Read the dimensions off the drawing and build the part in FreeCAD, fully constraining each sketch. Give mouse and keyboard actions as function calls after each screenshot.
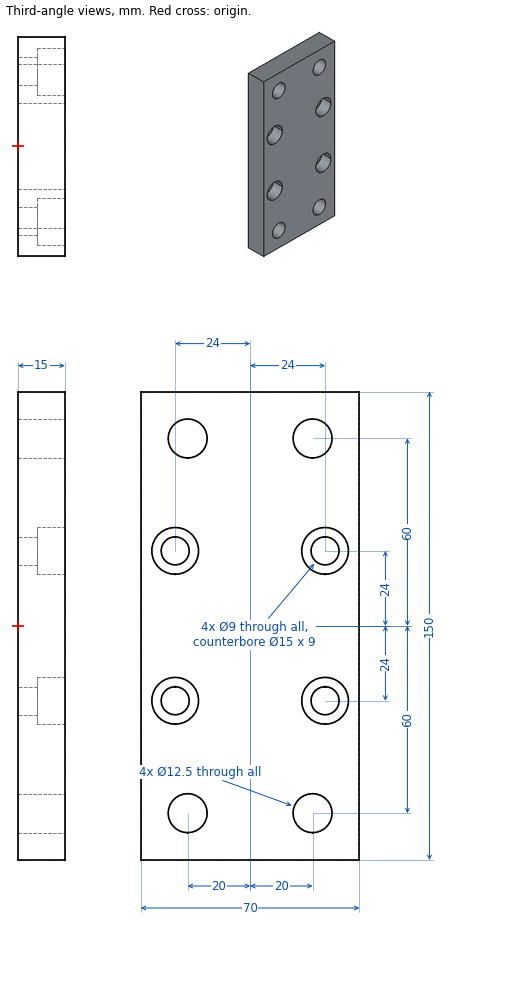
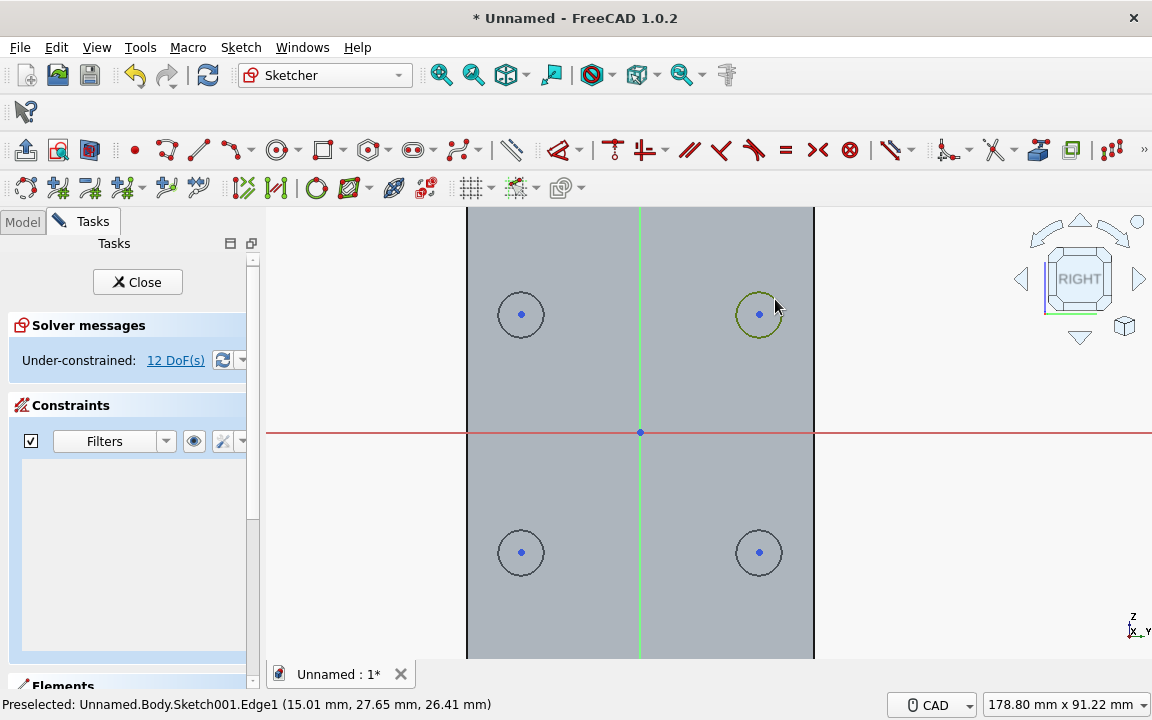
click(775, 537)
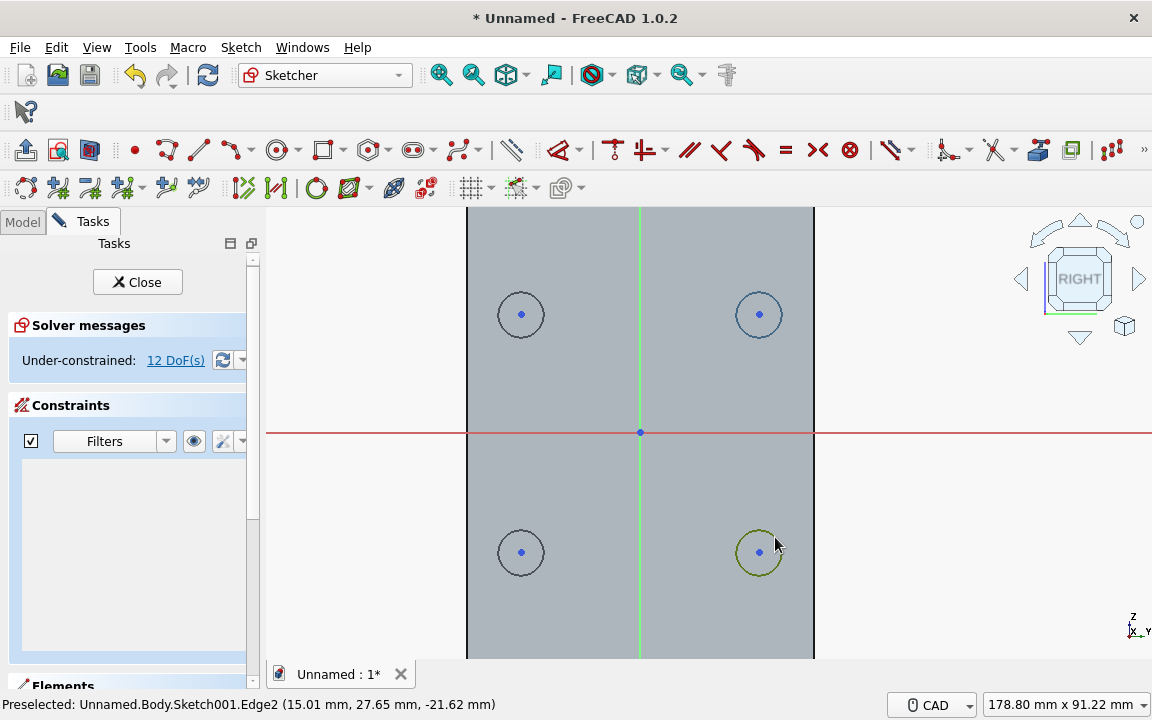
click(537, 299)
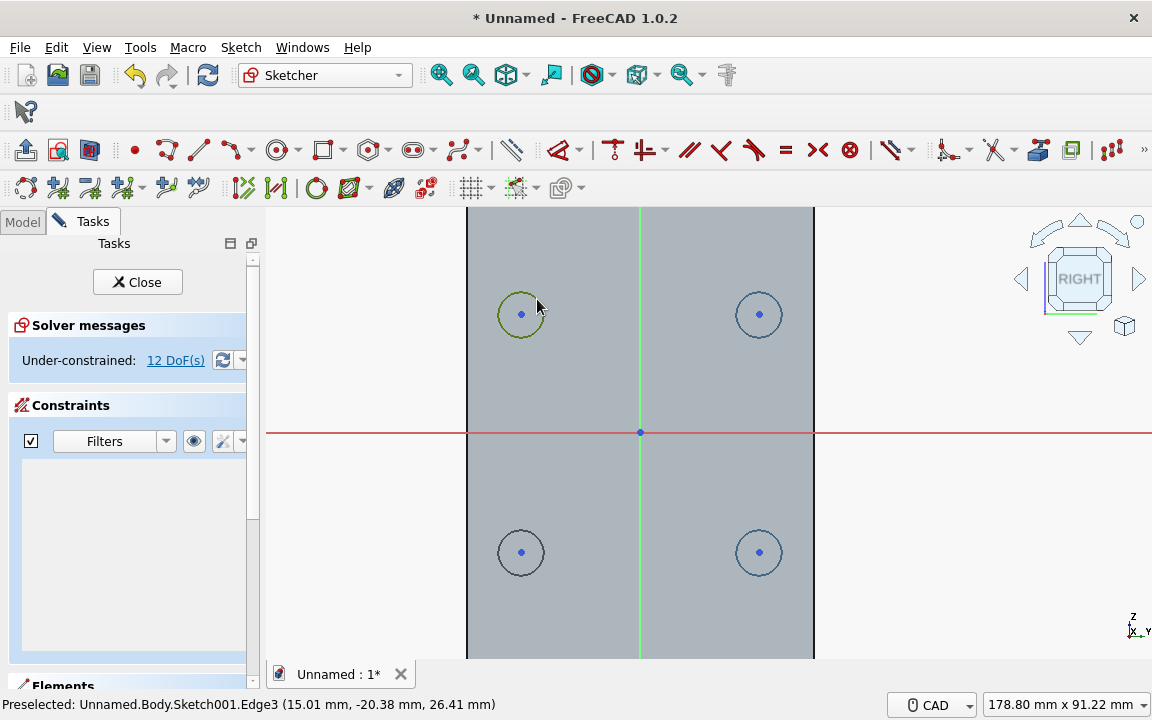
click(537, 537)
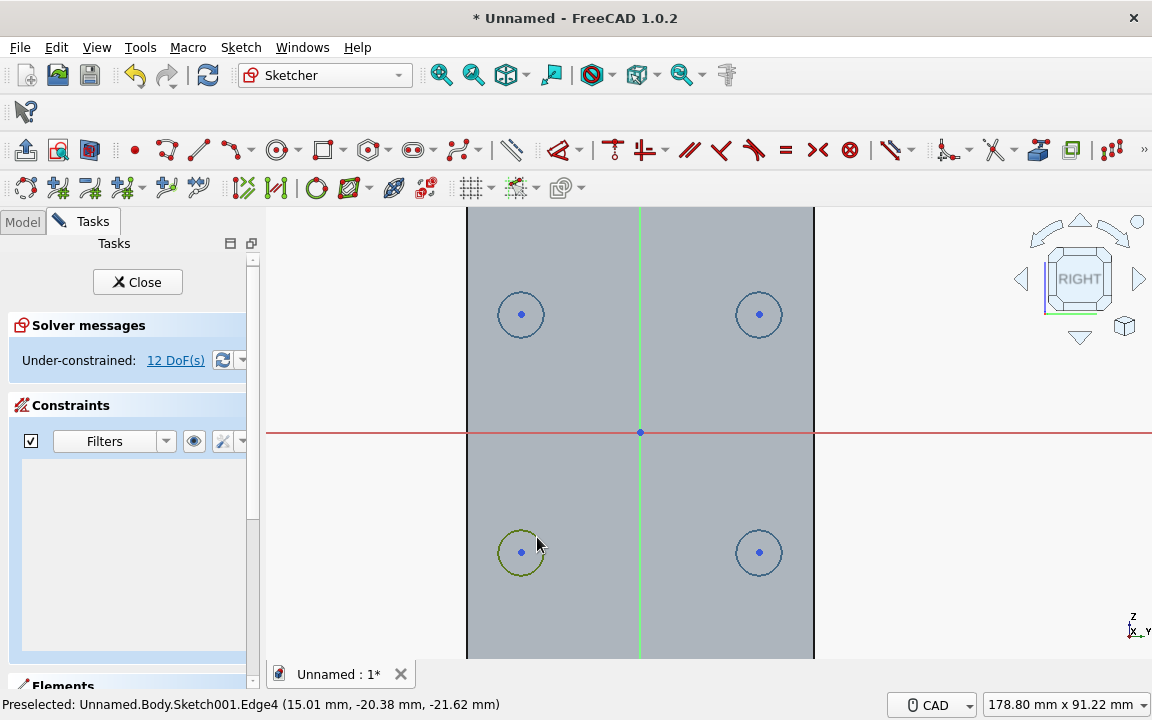
click(786, 150)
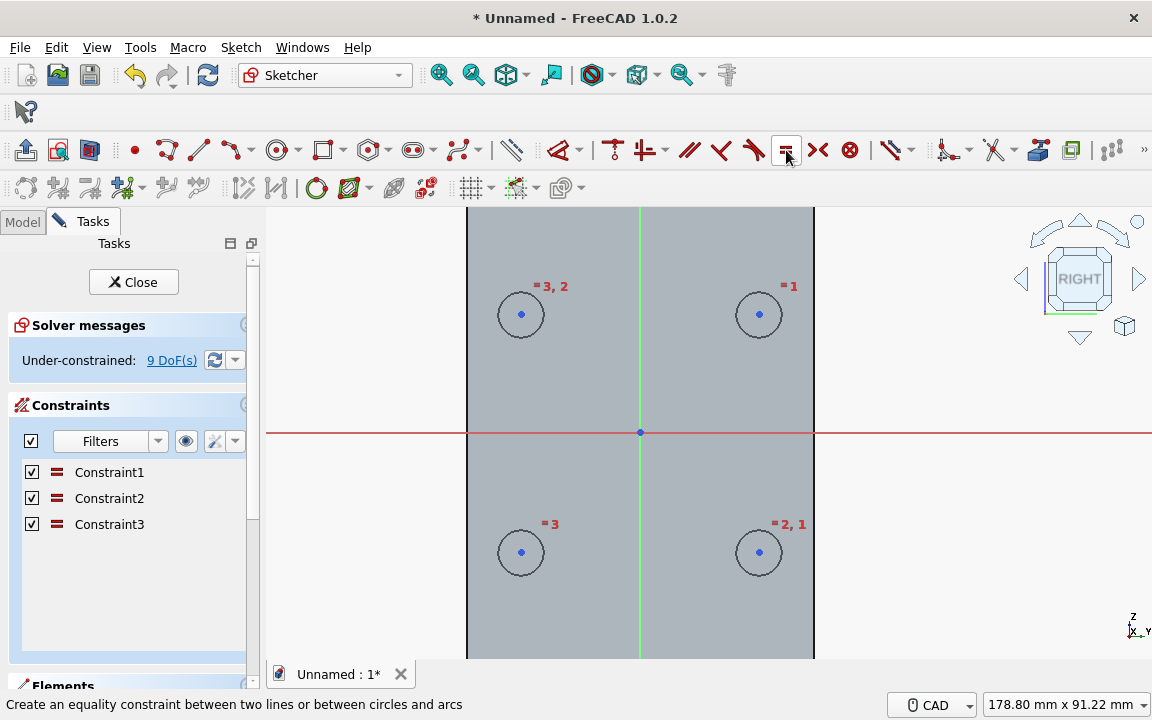
click(759, 315)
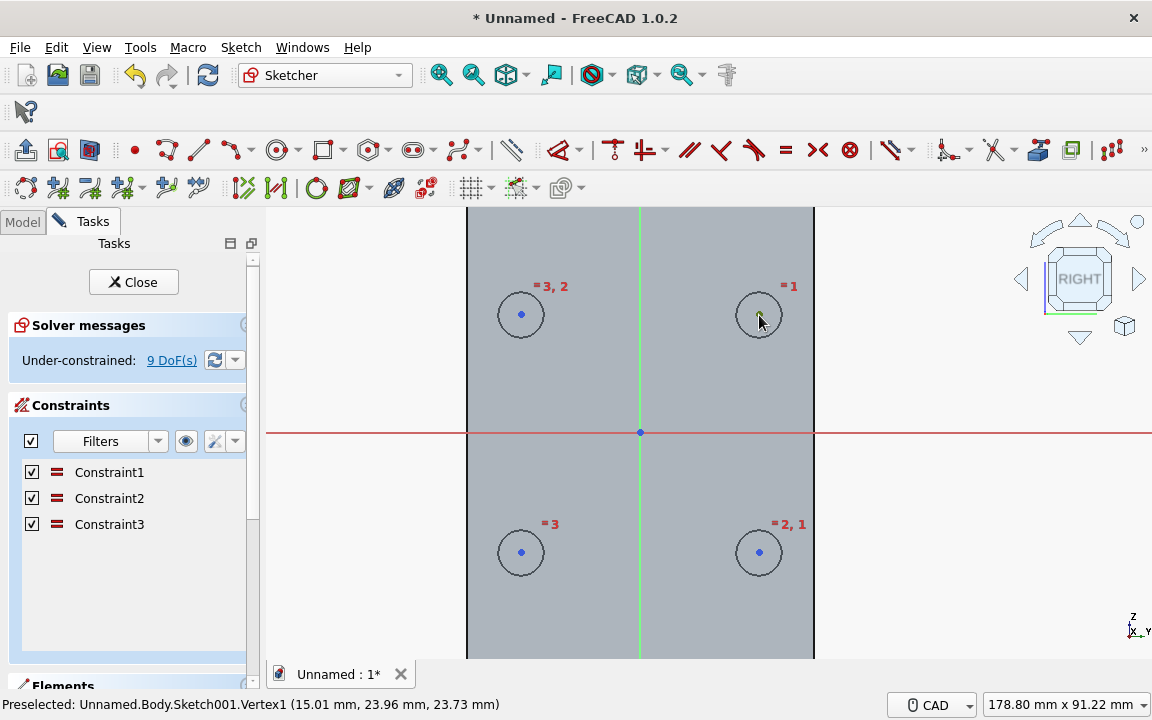
click(759, 553)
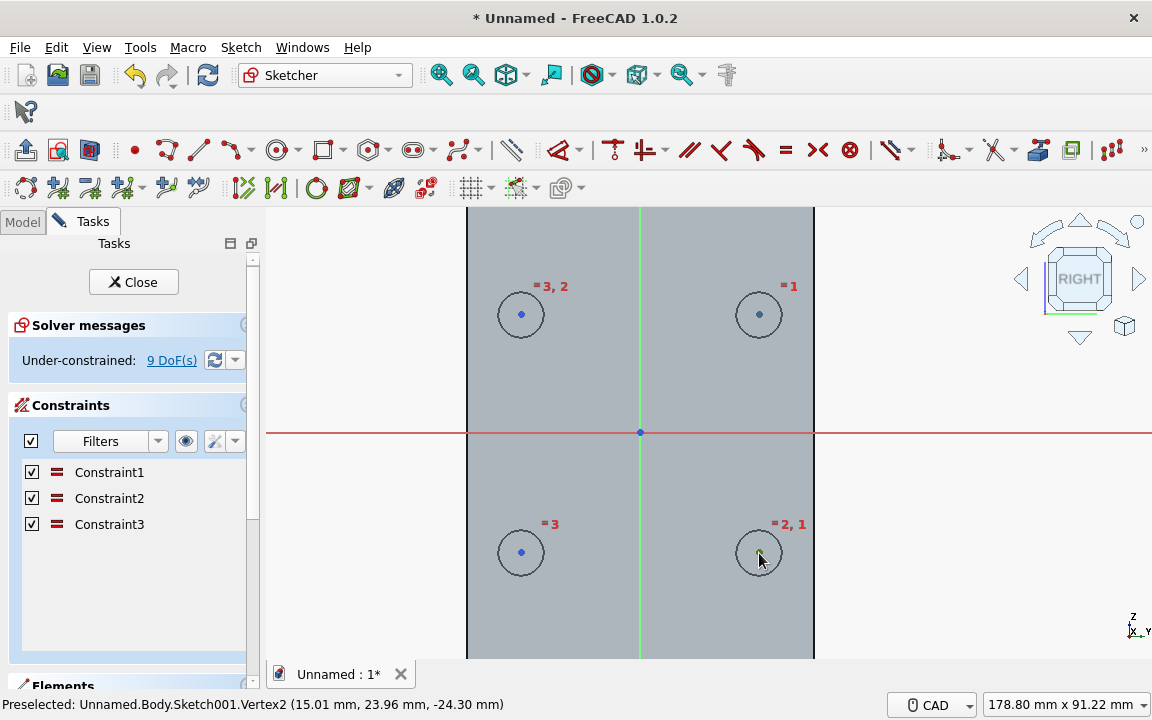
key(v)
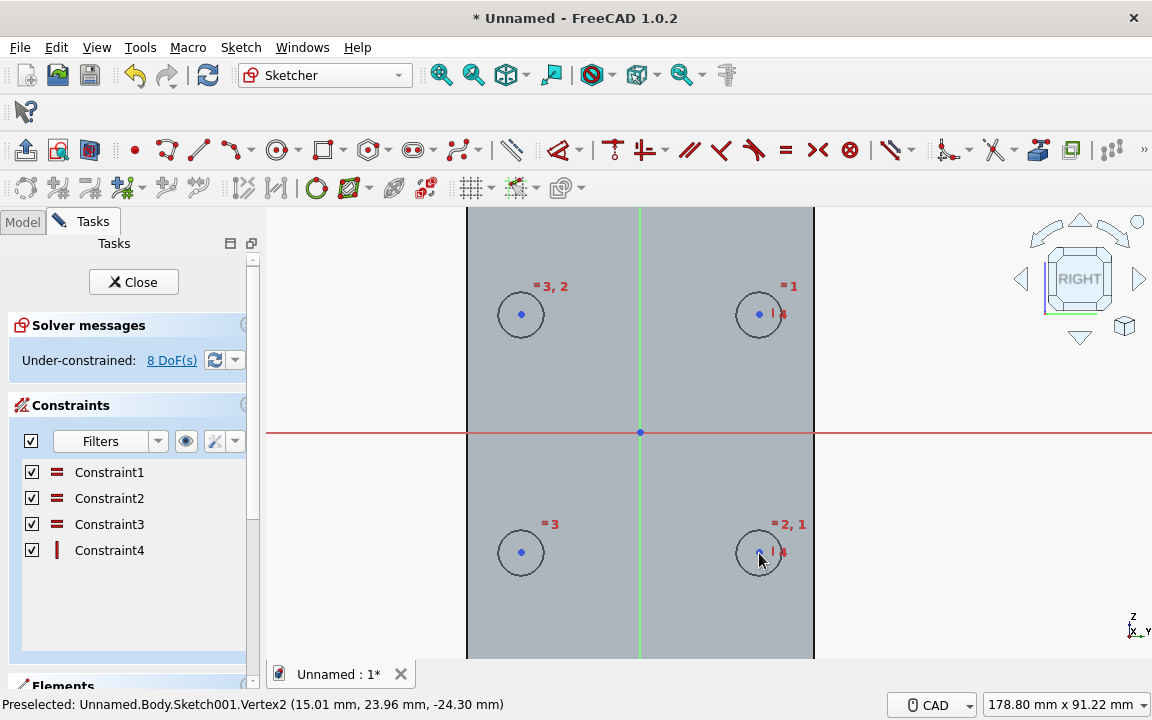
click(759, 315)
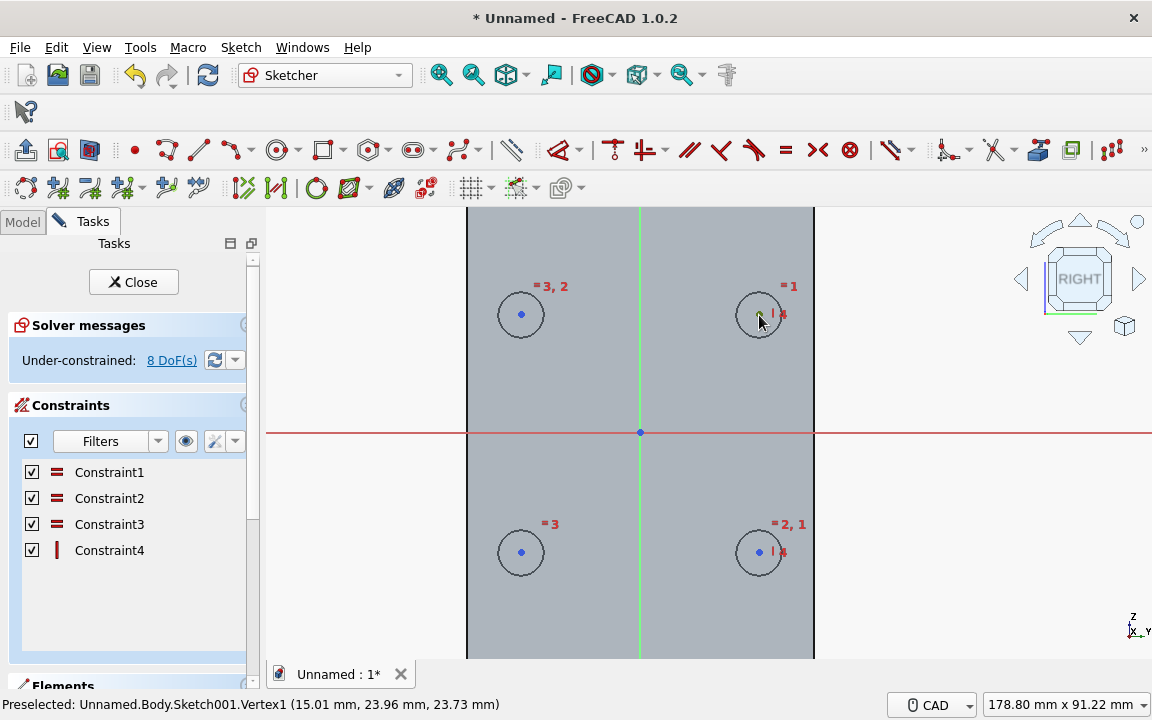
click(521, 315)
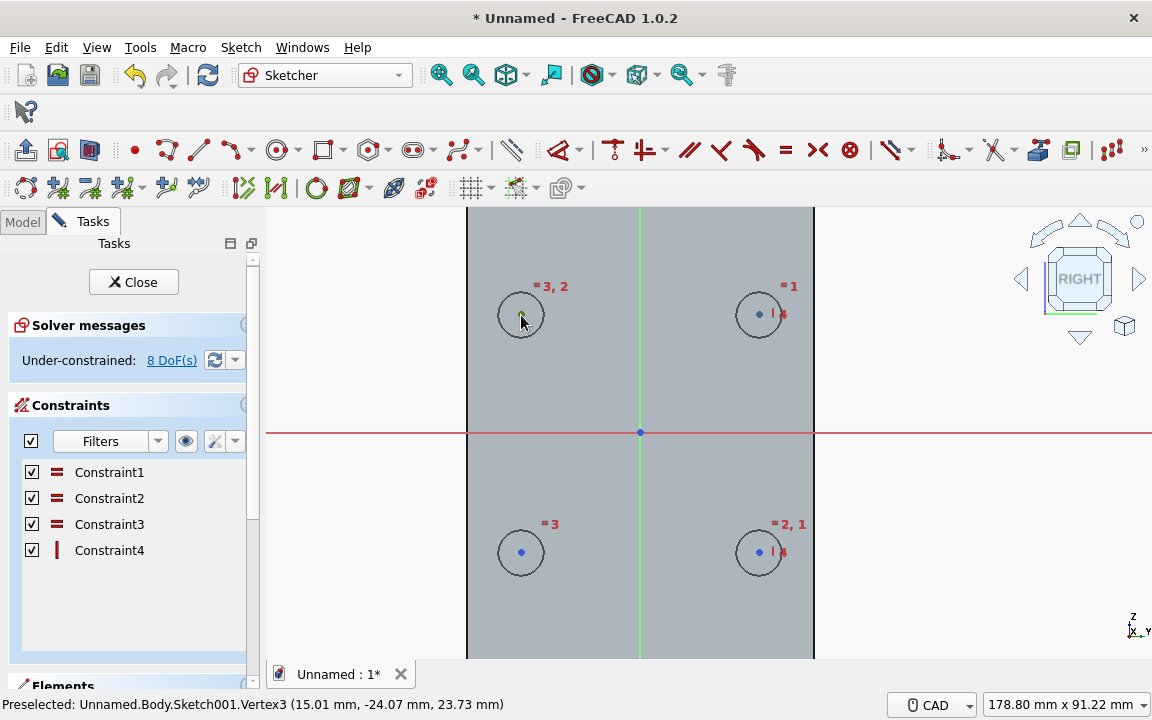
click(668, 150)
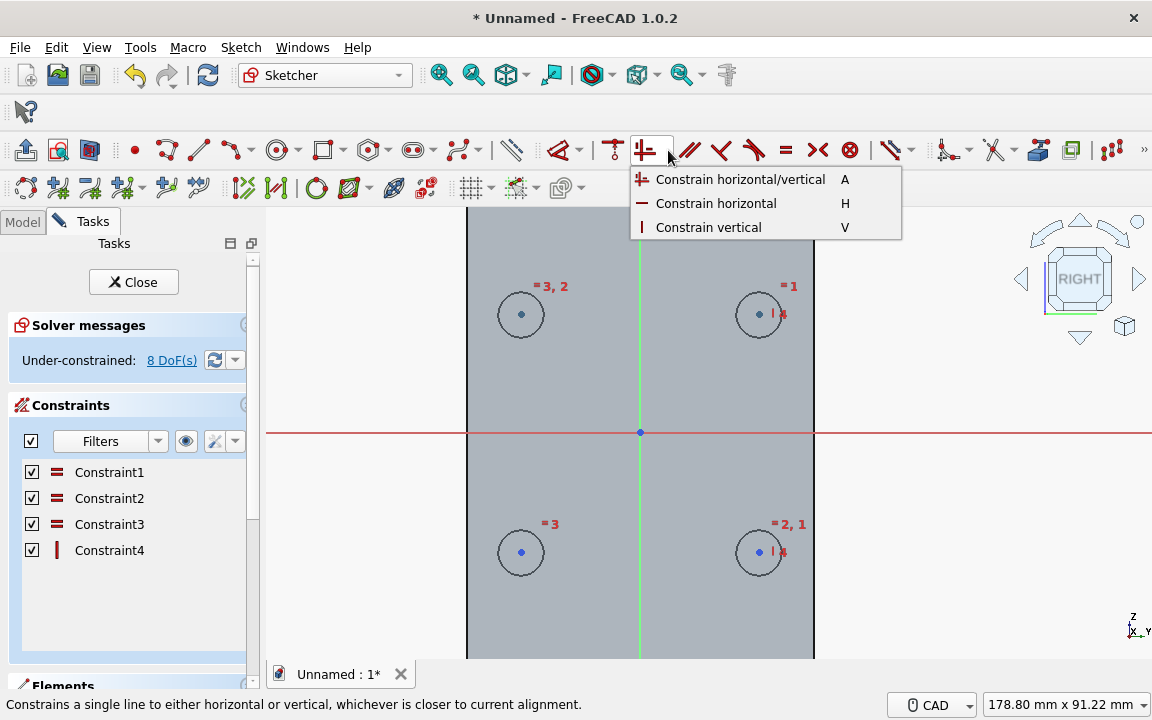
click(766, 203)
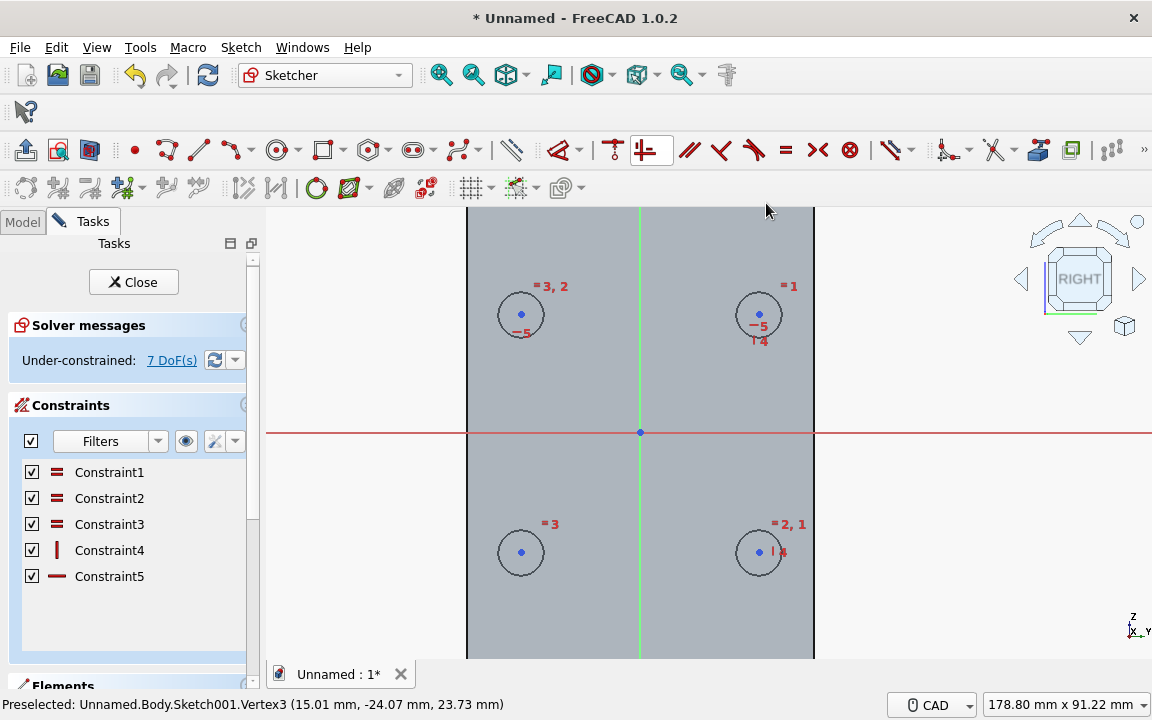
click(521, 315)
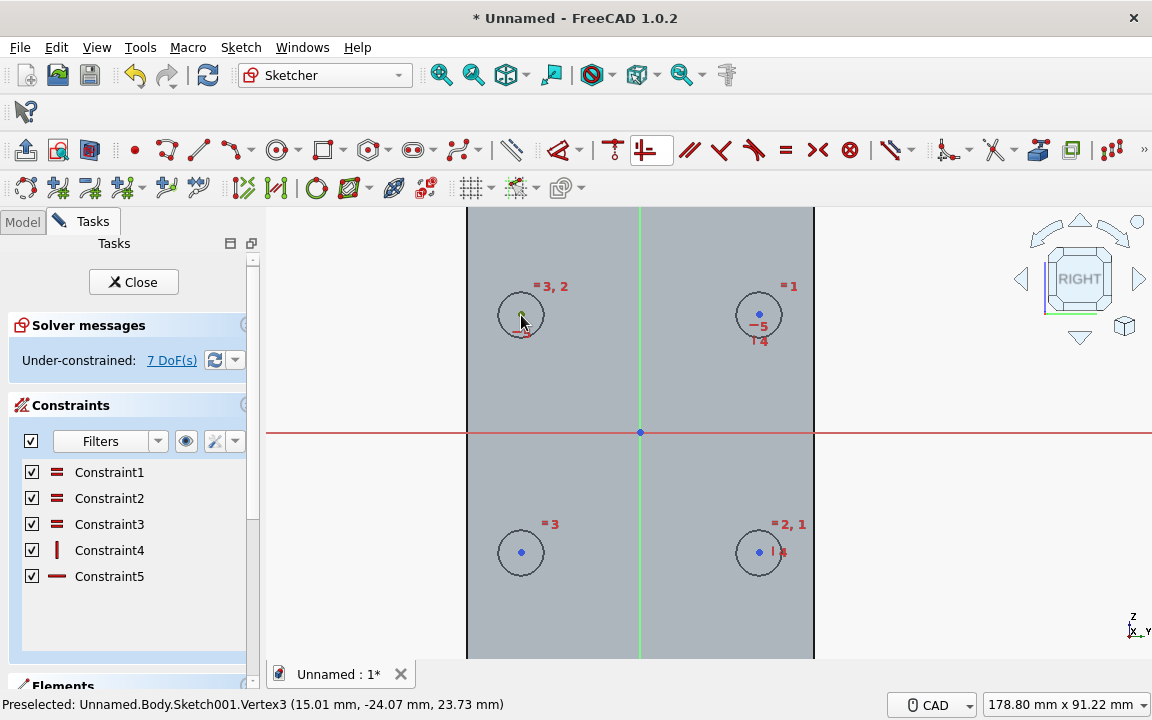
click(521, 553)